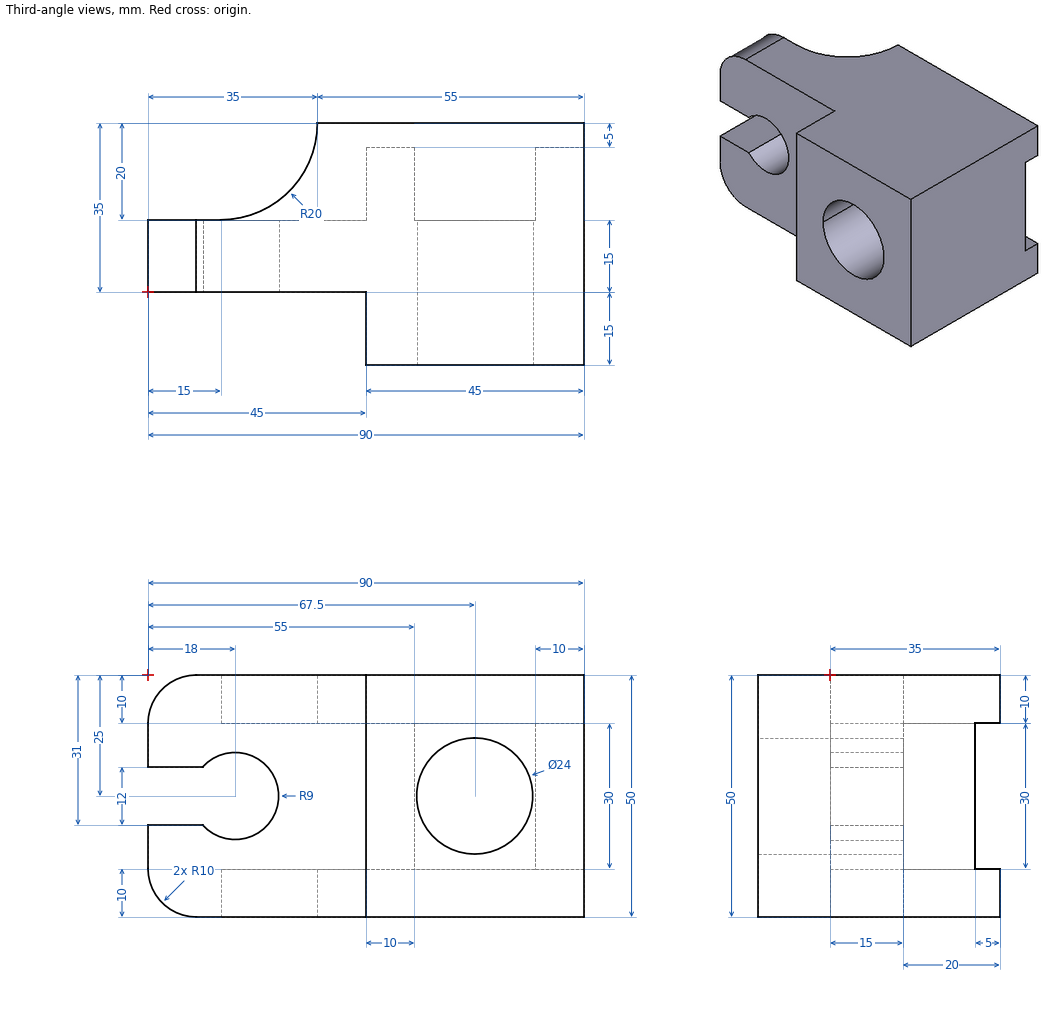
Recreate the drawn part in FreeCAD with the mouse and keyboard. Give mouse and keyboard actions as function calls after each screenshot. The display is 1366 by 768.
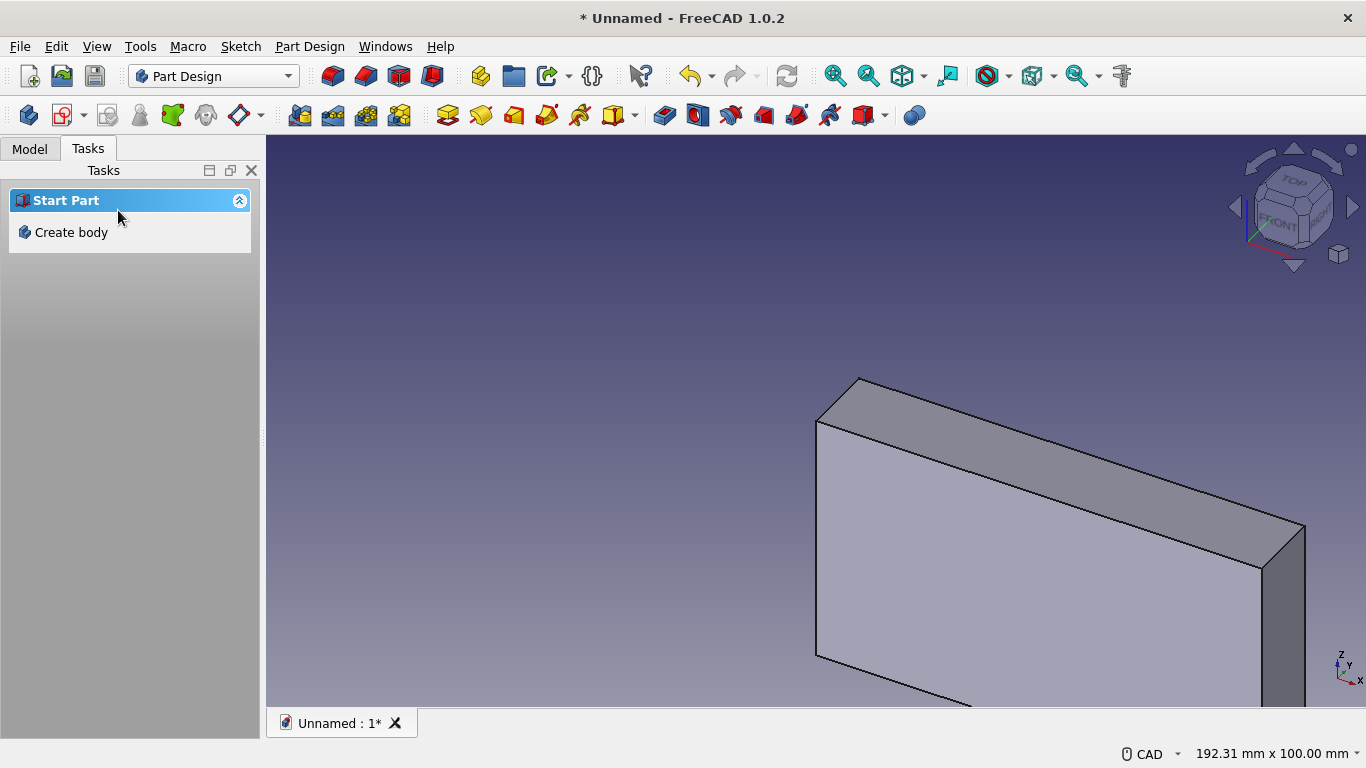
click(836, 76)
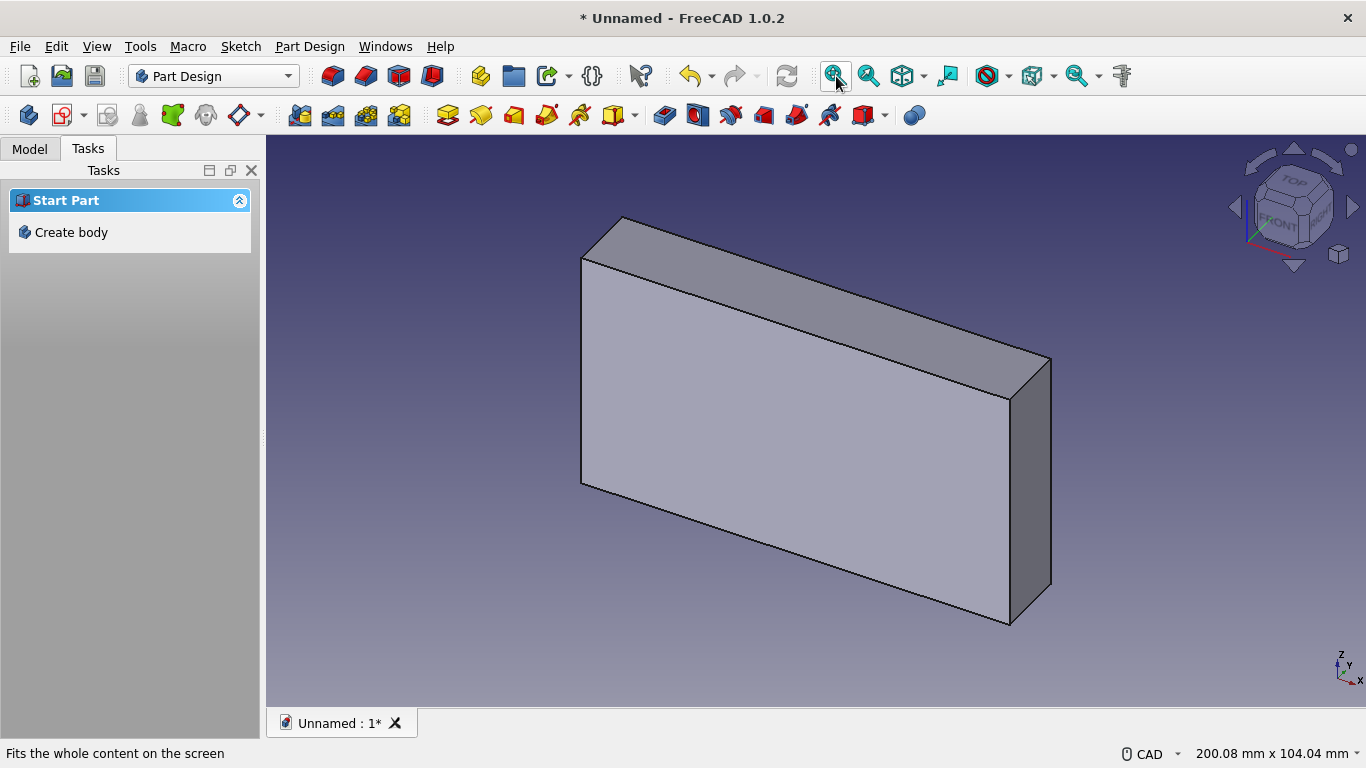
click(938, 348)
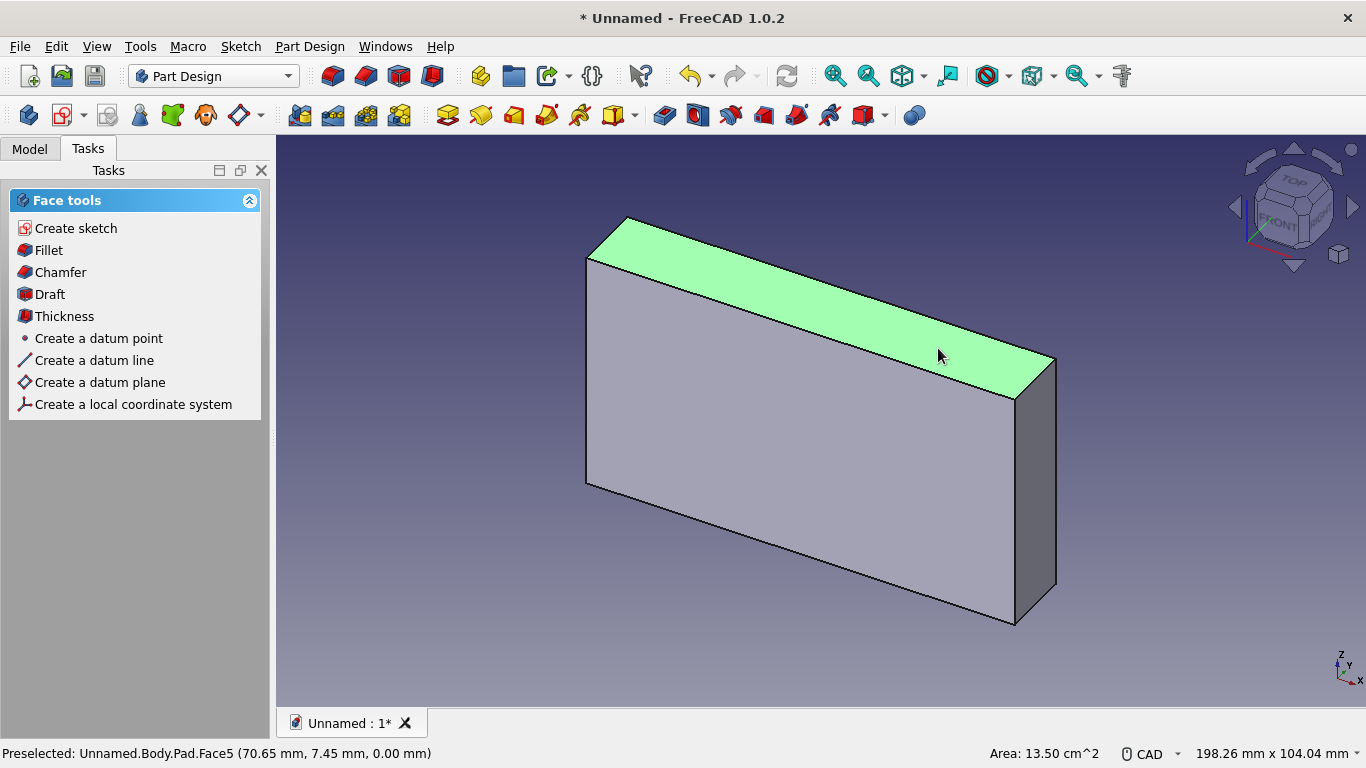
click(62, 116)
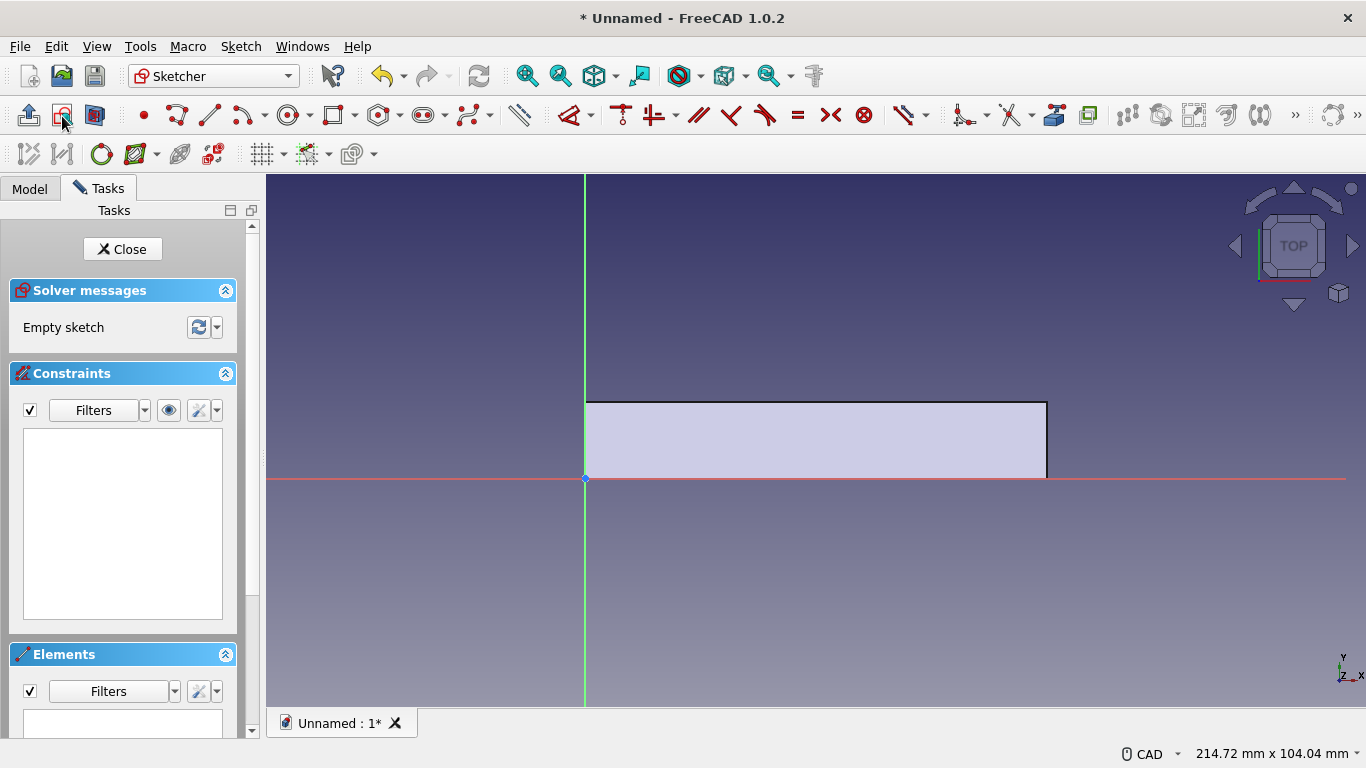
scroll(955, 674, up, 2)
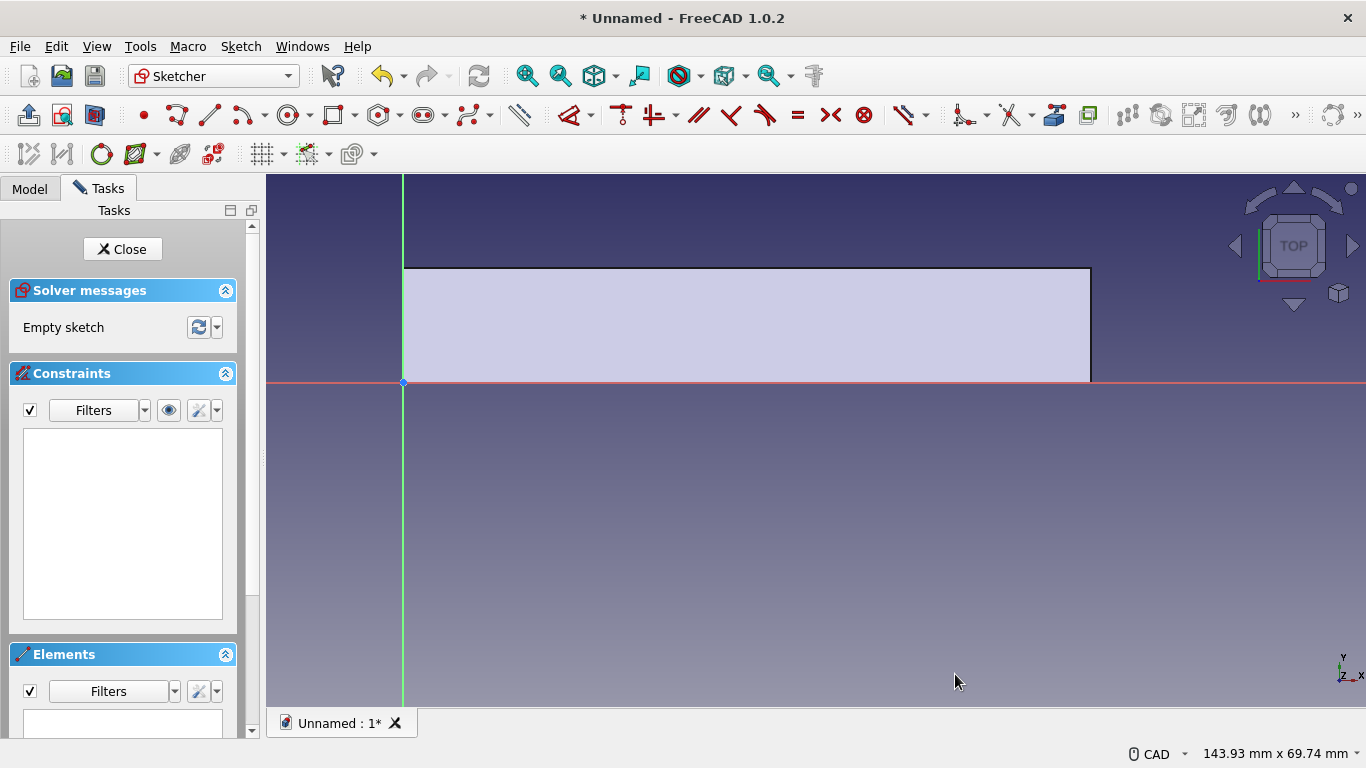
key(g)
key(r)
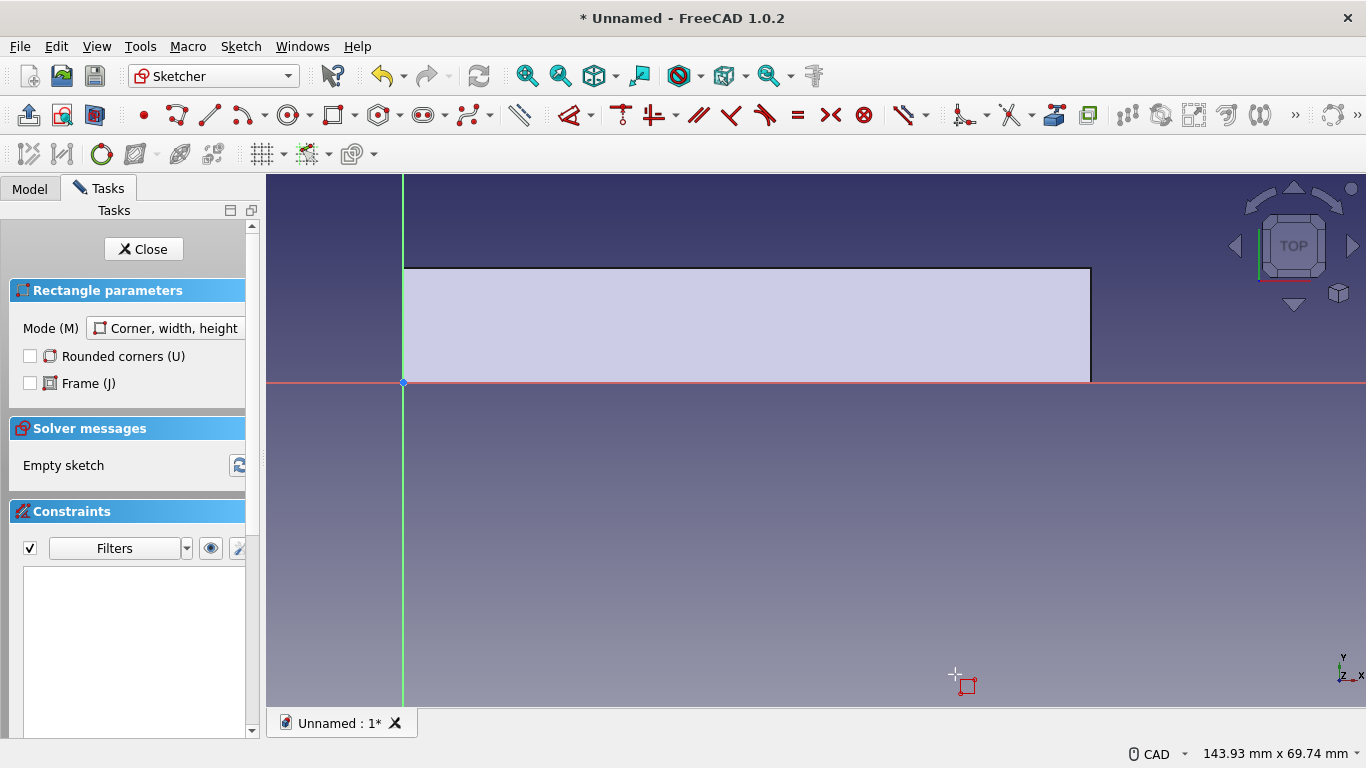
click(747, 383)
click(1091, 497)
key(Escape)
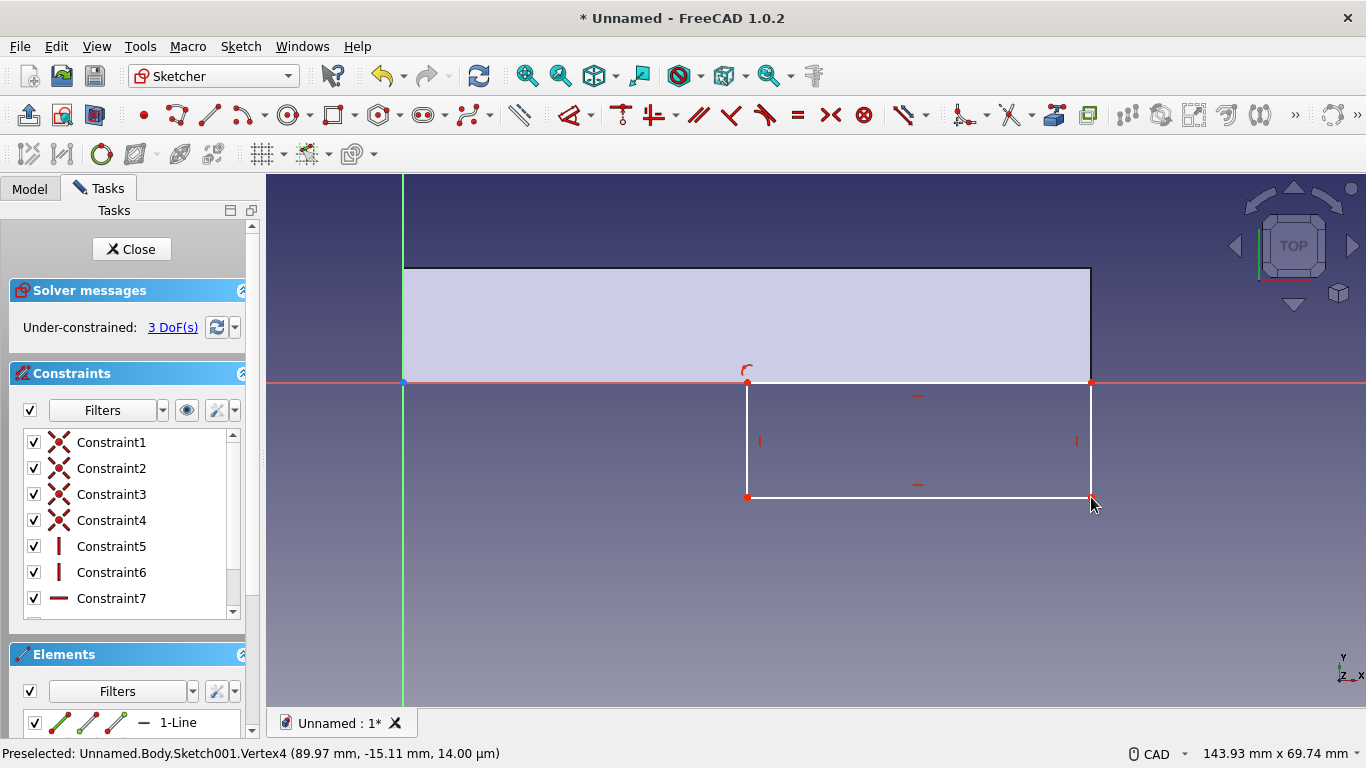
click(568, 116)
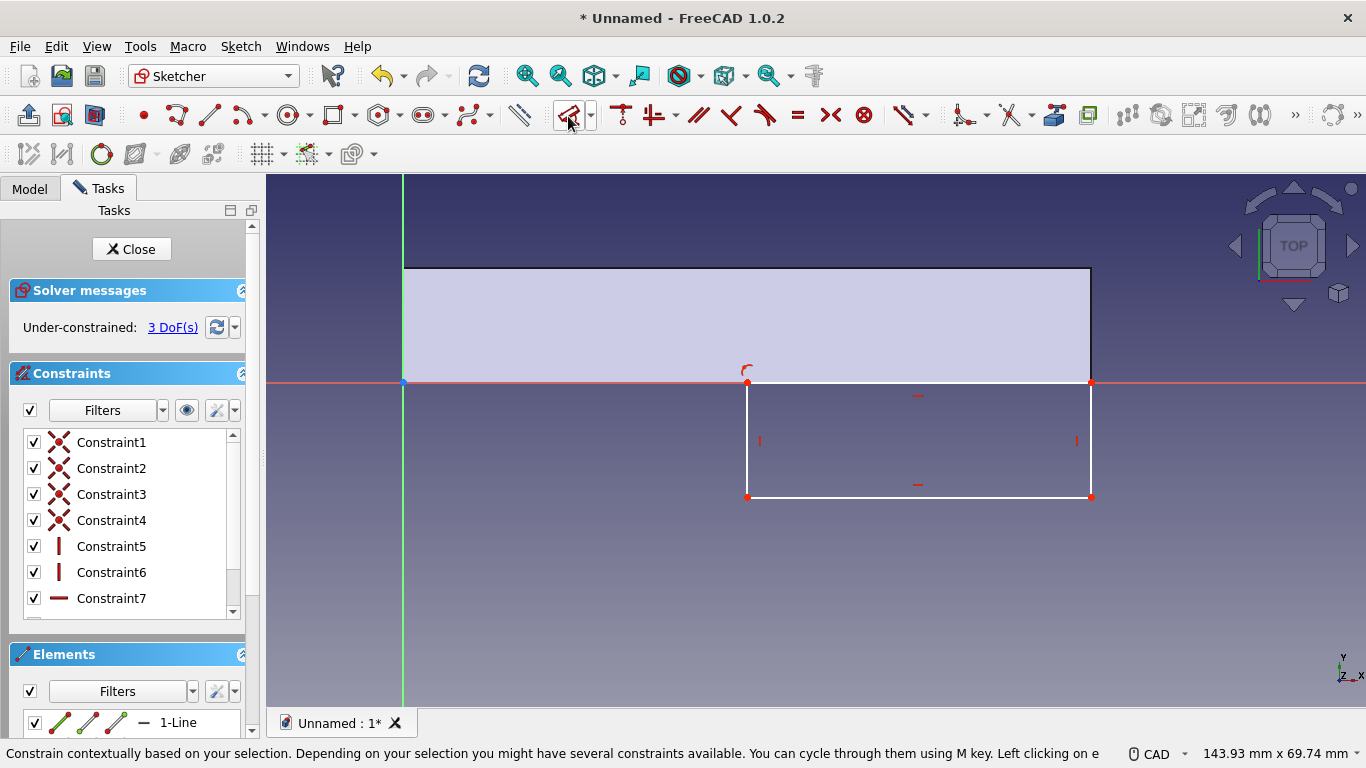
click(747, 417)
click(713, 440)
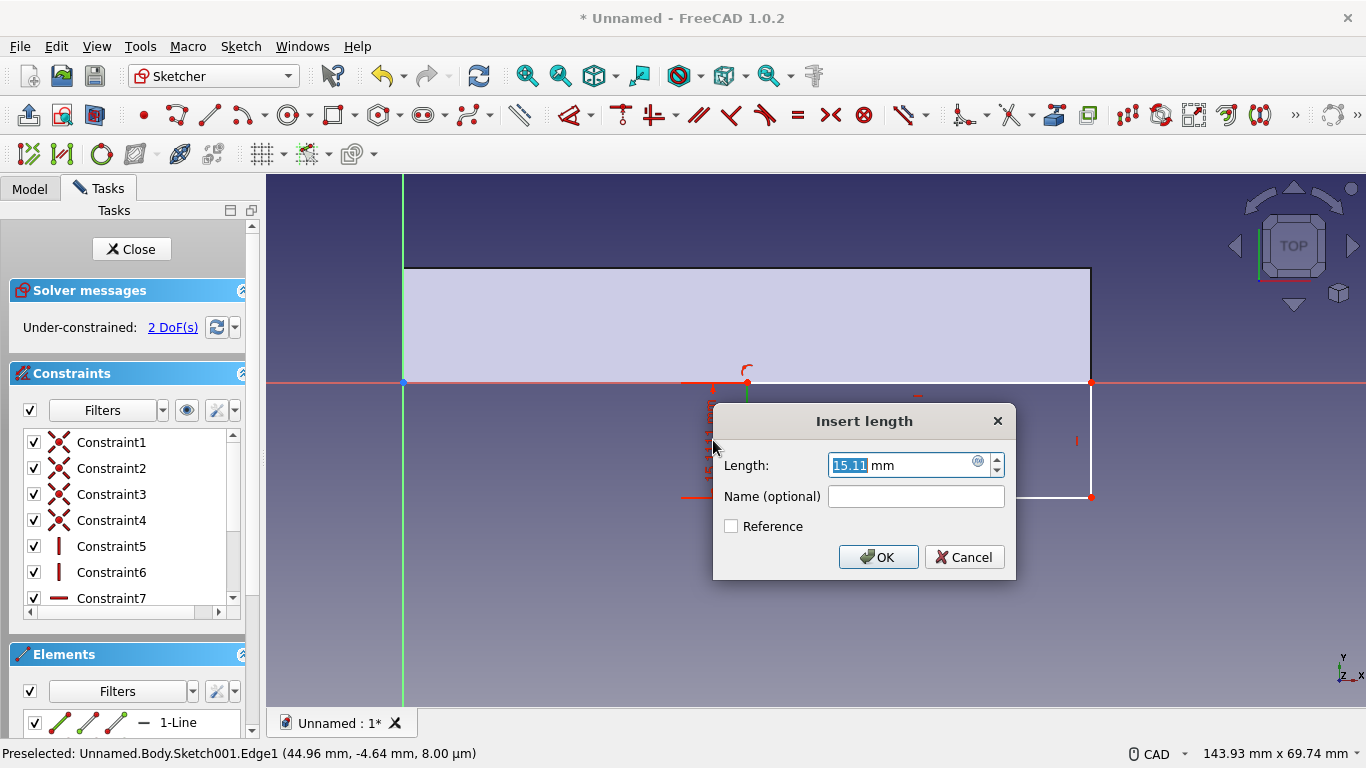
text(15)
key(Return)